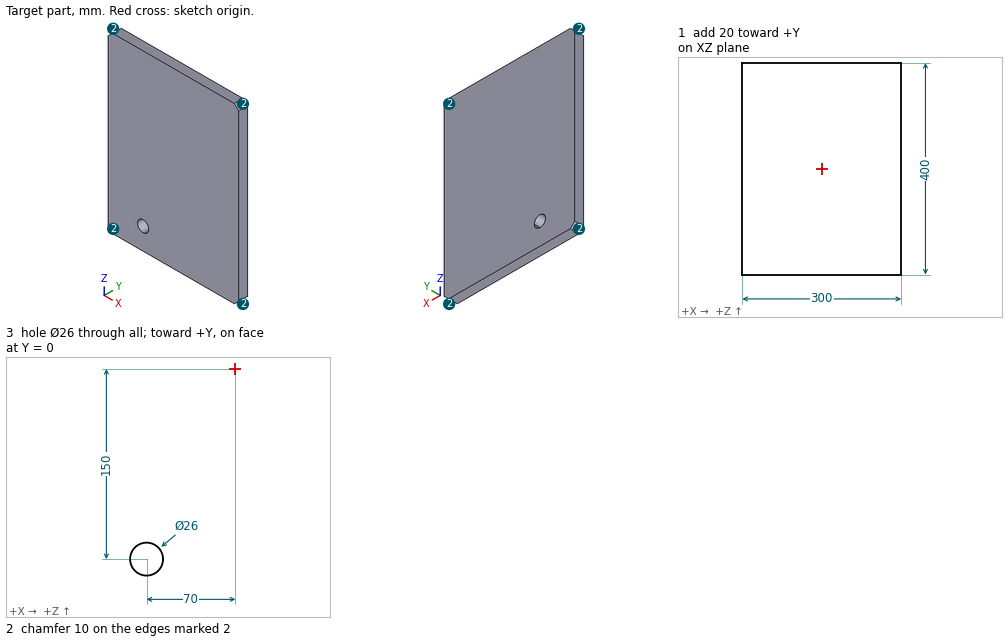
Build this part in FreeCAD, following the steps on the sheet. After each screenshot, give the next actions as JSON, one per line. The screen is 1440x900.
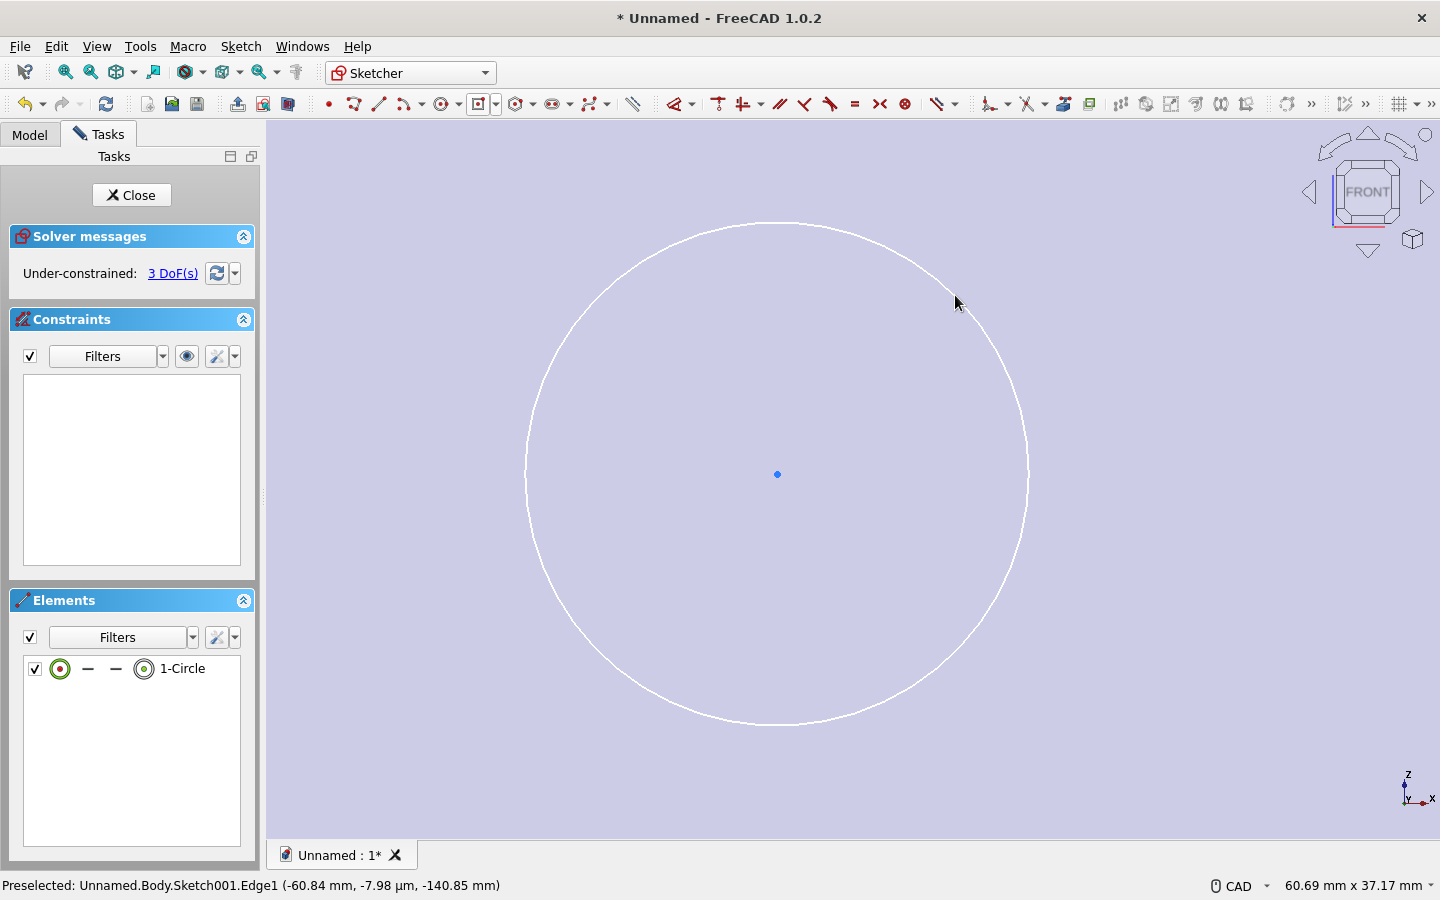
{"action": "left_click", "coordinate": [674, 104]}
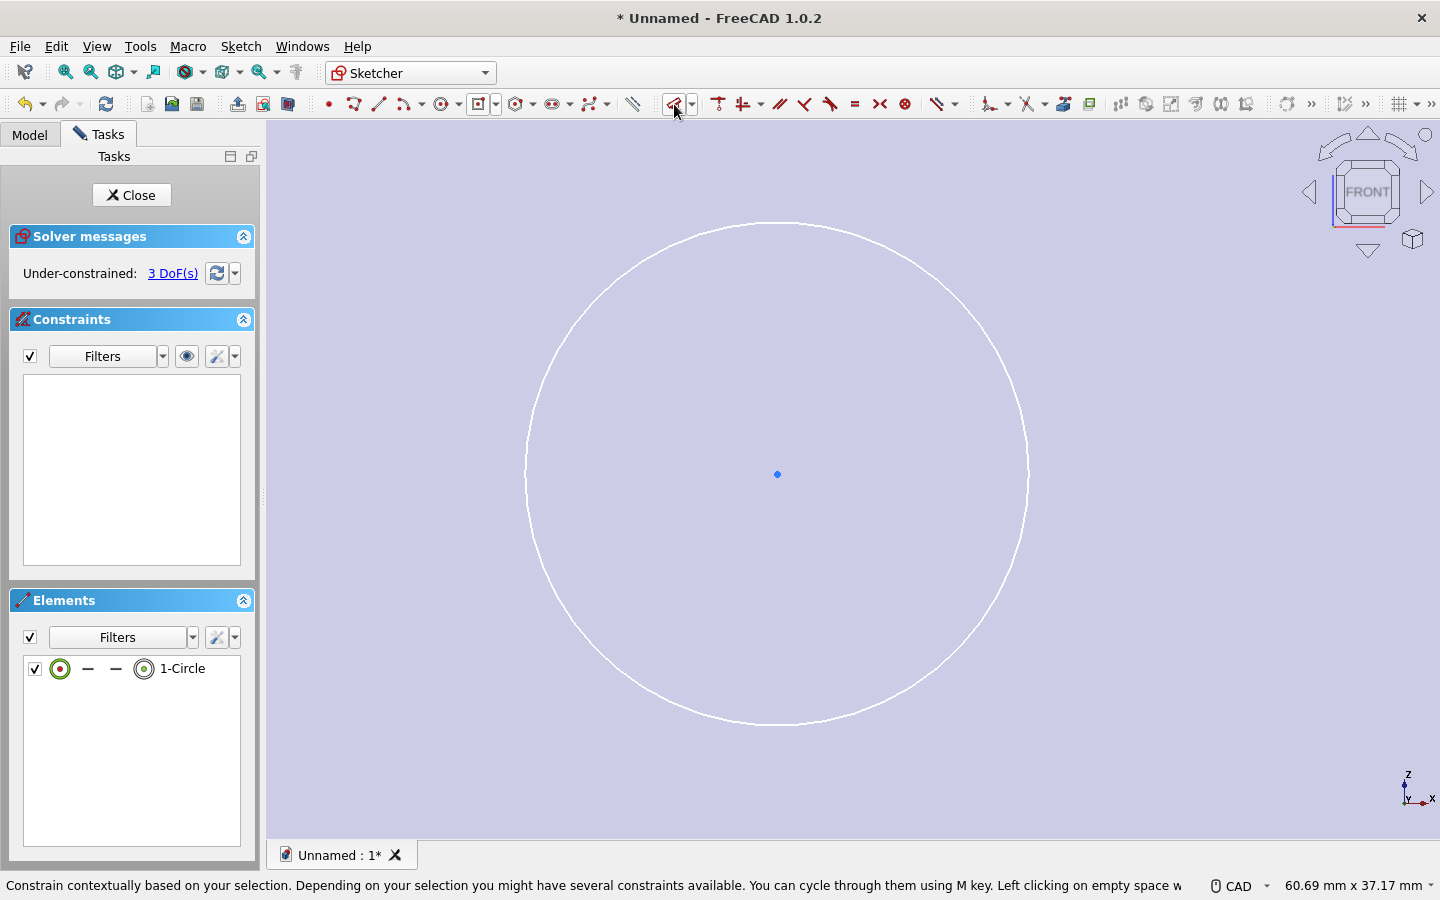
{"action": "left_click", "coordinate": [954, 295]}
{"action": "left_click", "coordinate": [976, 272]}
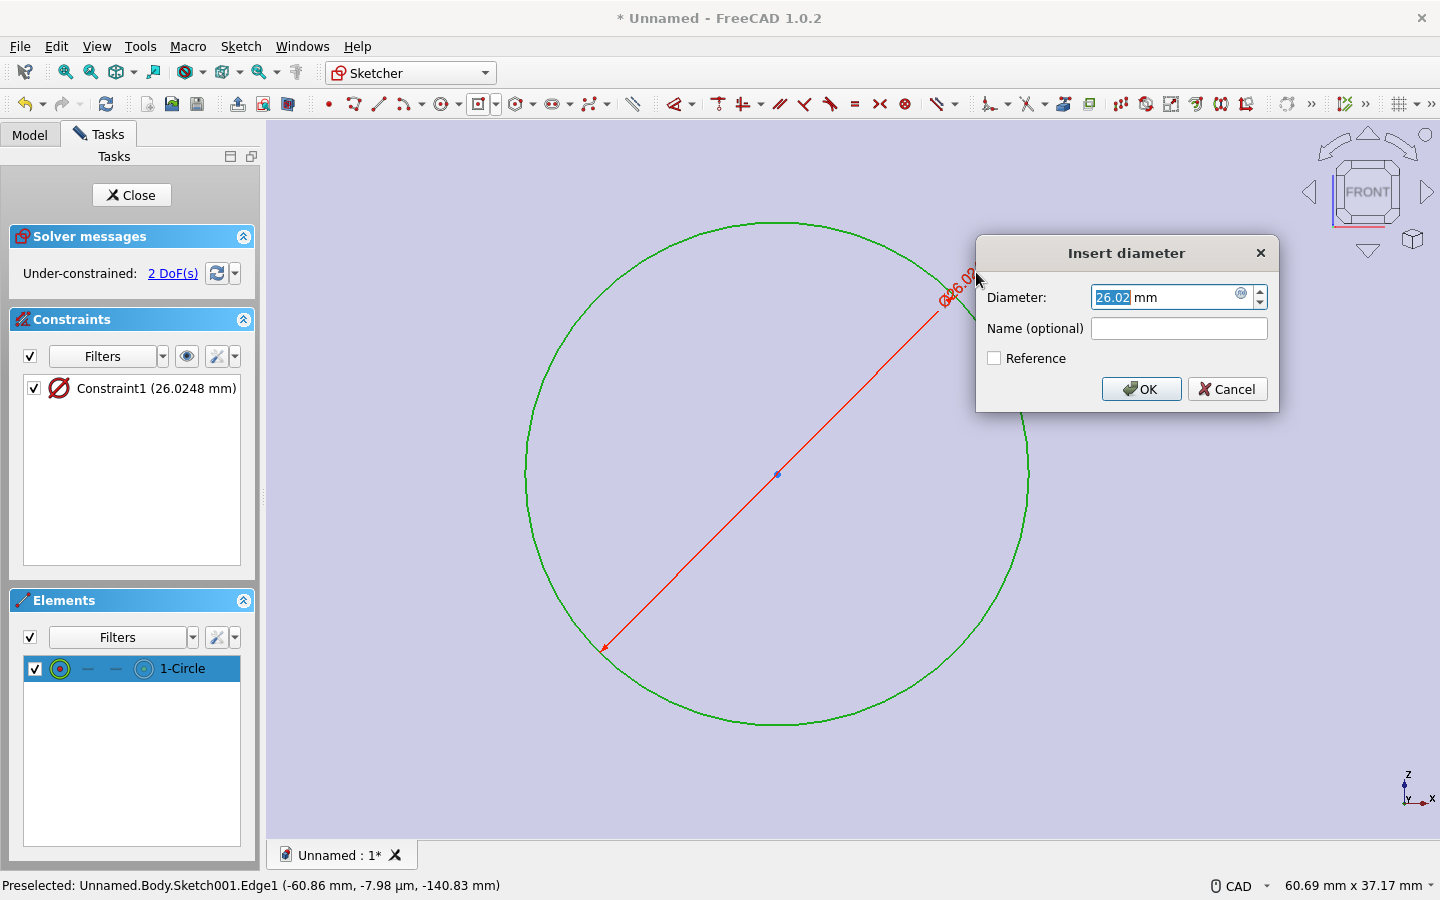
{"action": "type", "text": "26"}
{"action": "key", "text": "Return"}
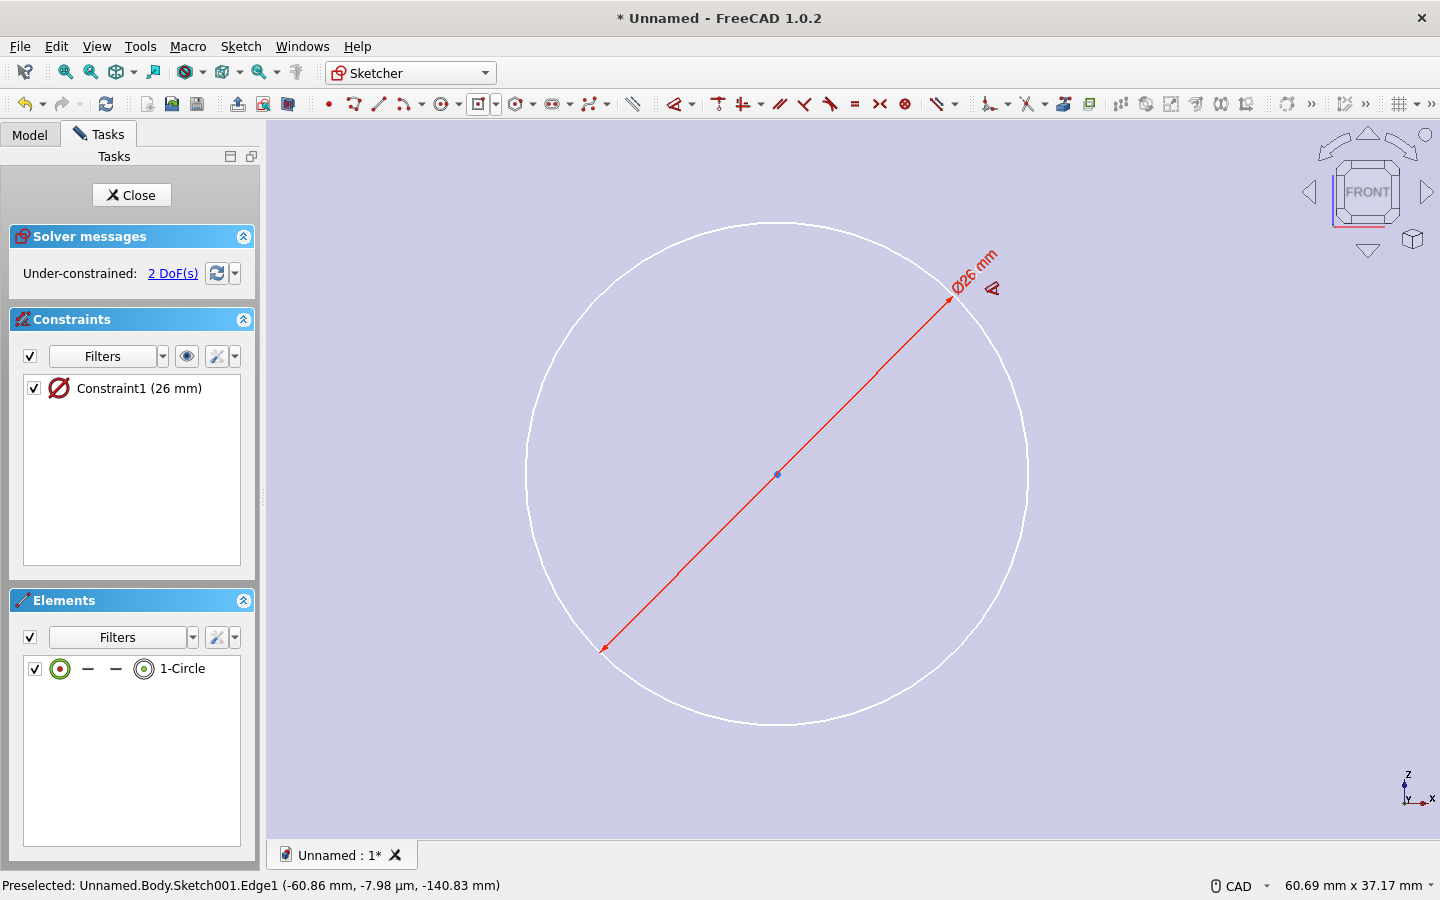
{"action": "left_click", "coordinate": [777, 474]}
{"action": "left_click", "coordinate": [911, 508]}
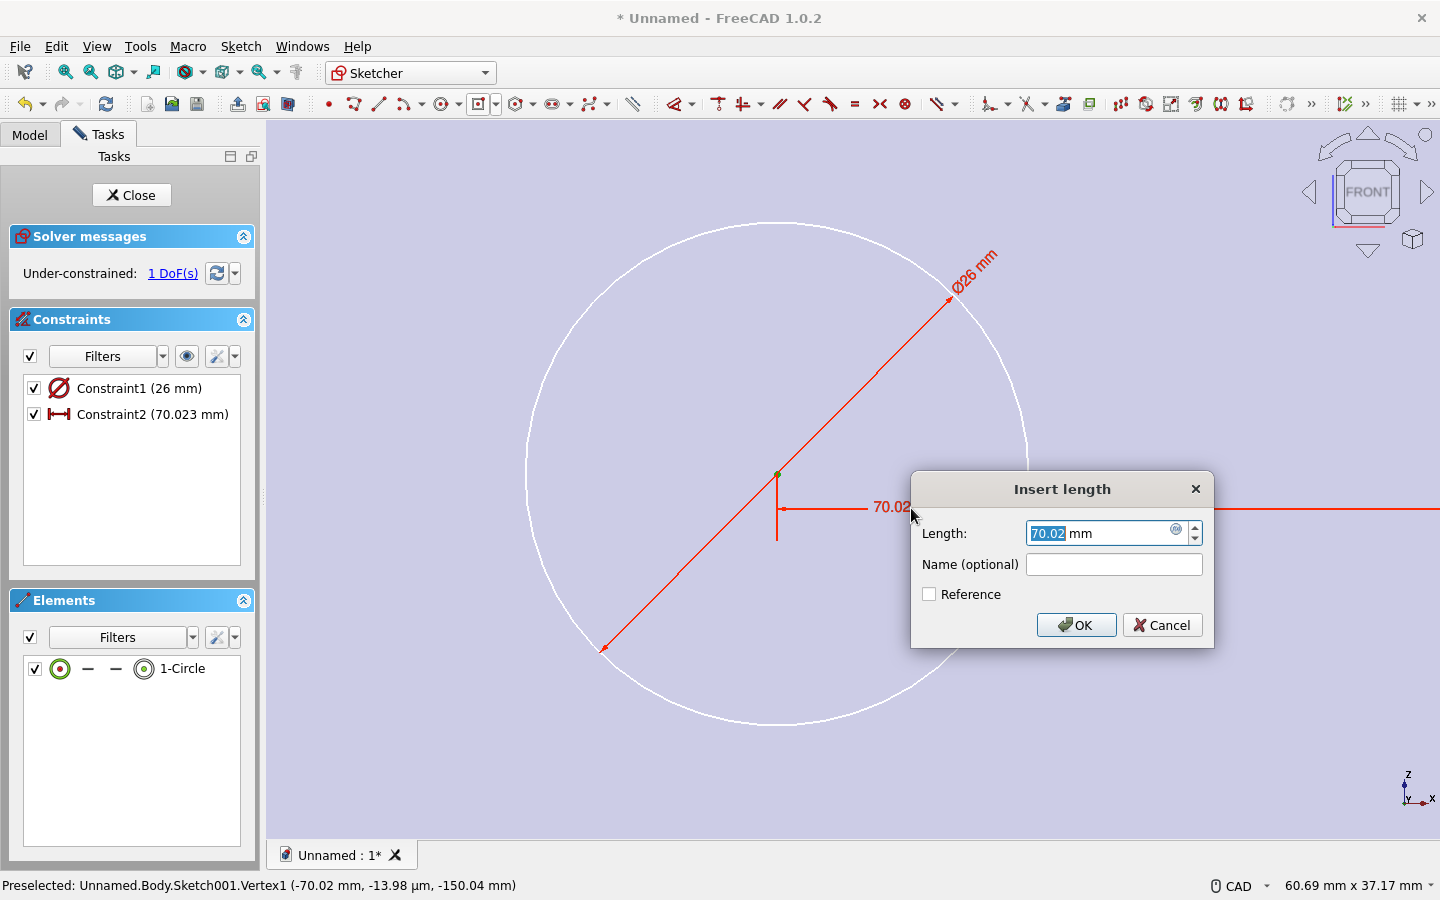
{"action": "type", "text": "70"}
{"action": "key", "text": "Return"}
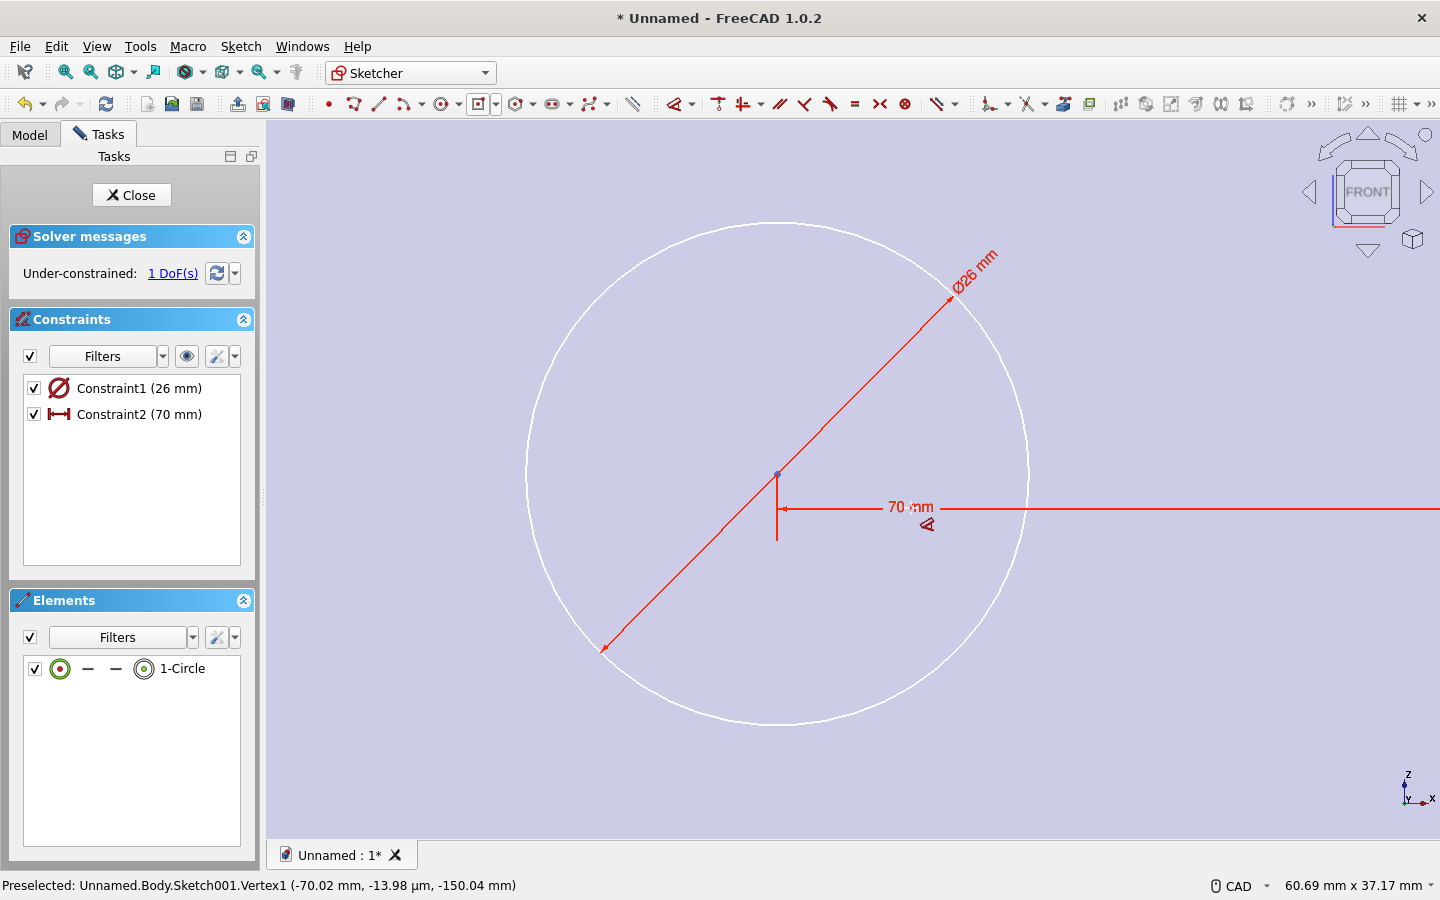
{"action": "left_click", "coordinate": [777, 474]}
{"action": "left_click", "coordinate": [743, 311]}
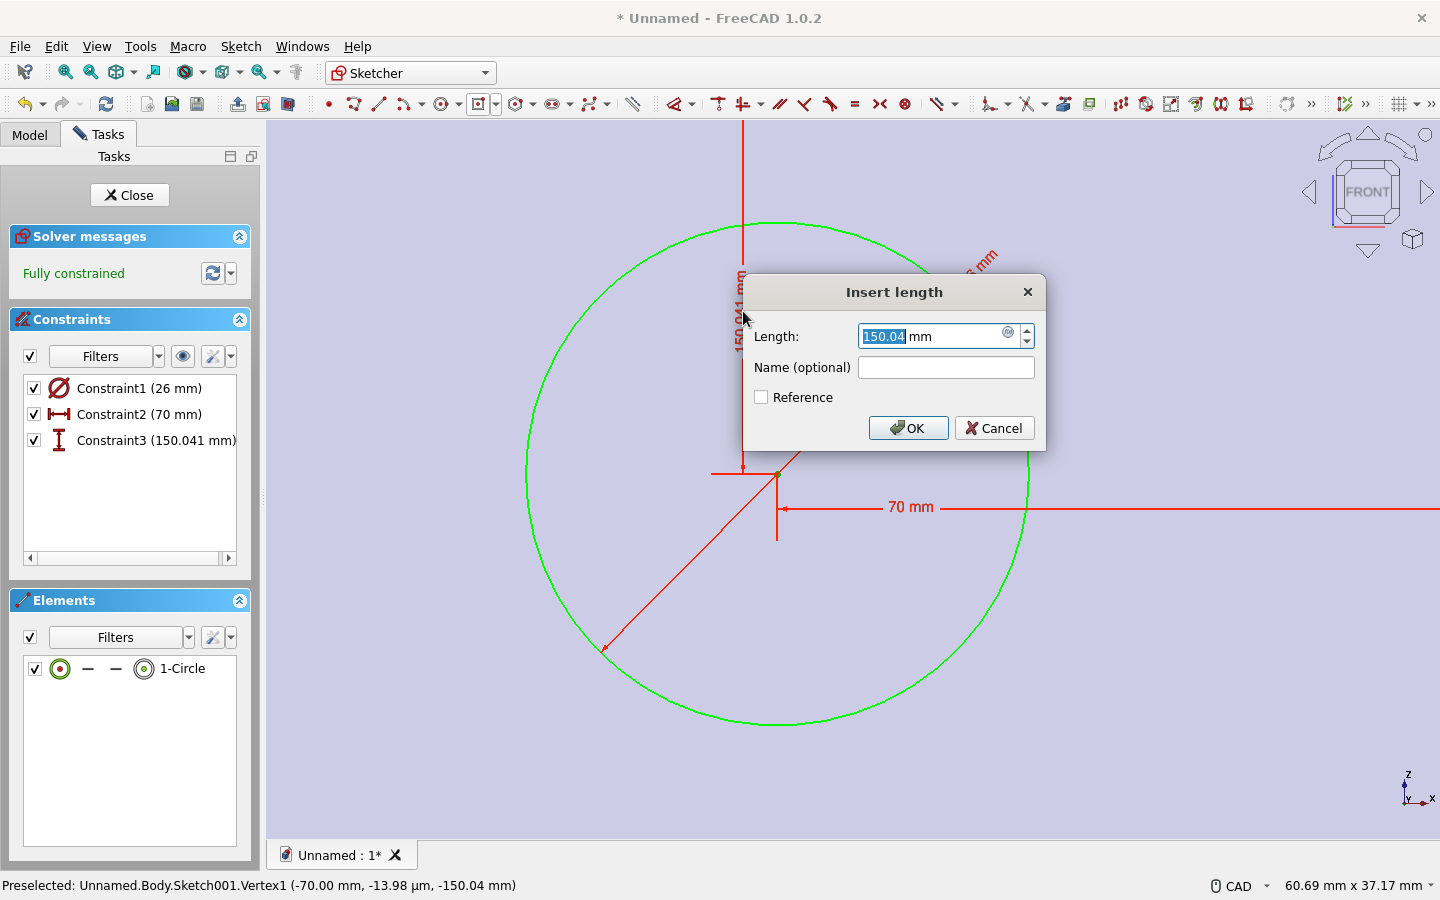
{"action": "type", "text": "150"}
{"action": "key", "text": "Return"}
{"action": "key", "text": "Escape"}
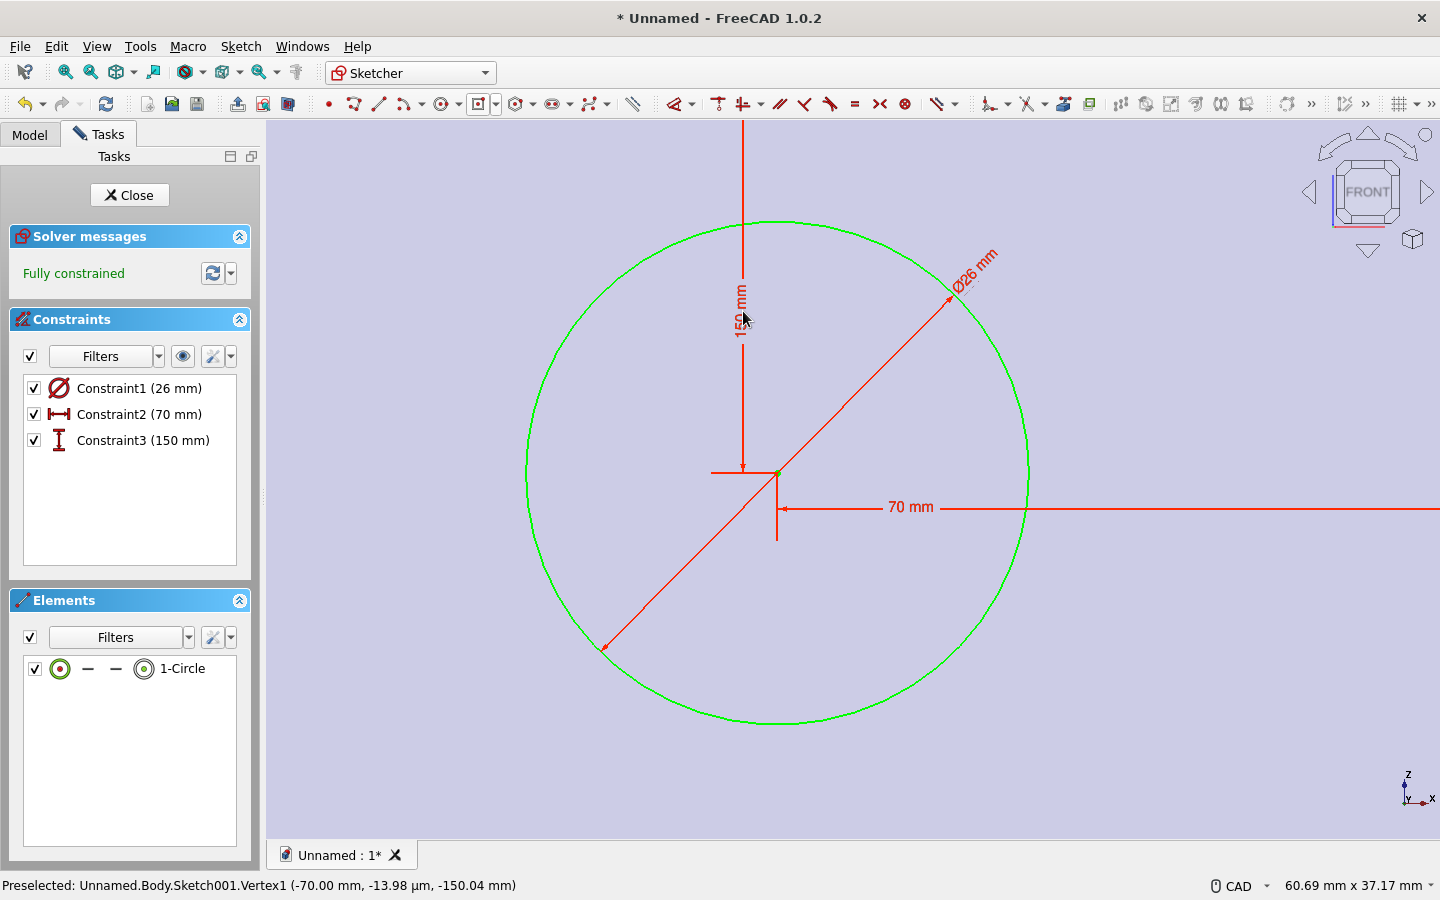
{"action": "left_click", "coordinate": [130, 195]}